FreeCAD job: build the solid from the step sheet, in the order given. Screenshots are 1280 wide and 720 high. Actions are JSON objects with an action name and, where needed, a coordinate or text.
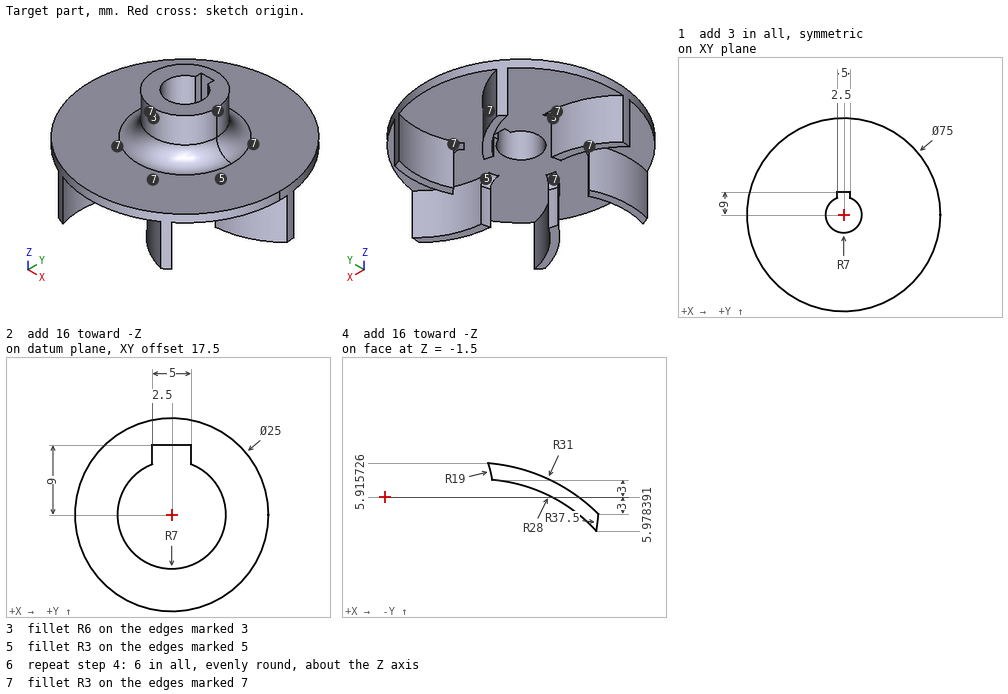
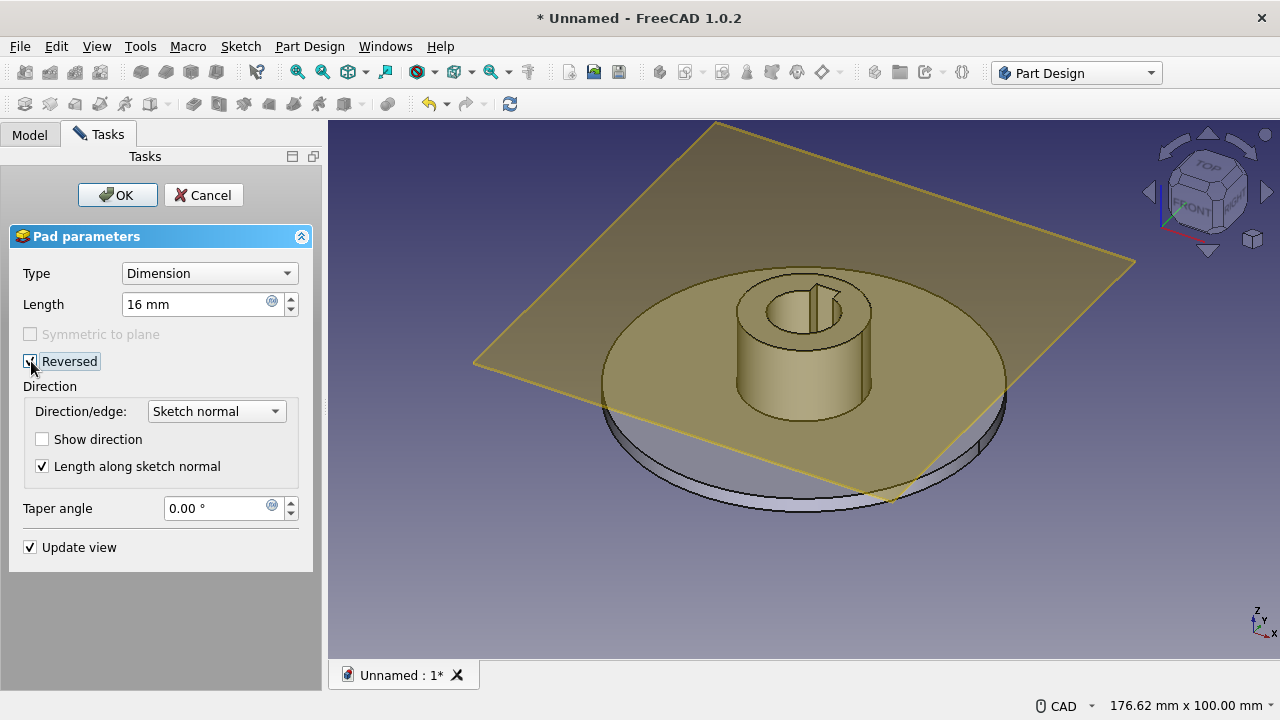
{"action": "left_click", "coordinate": [118, 195]}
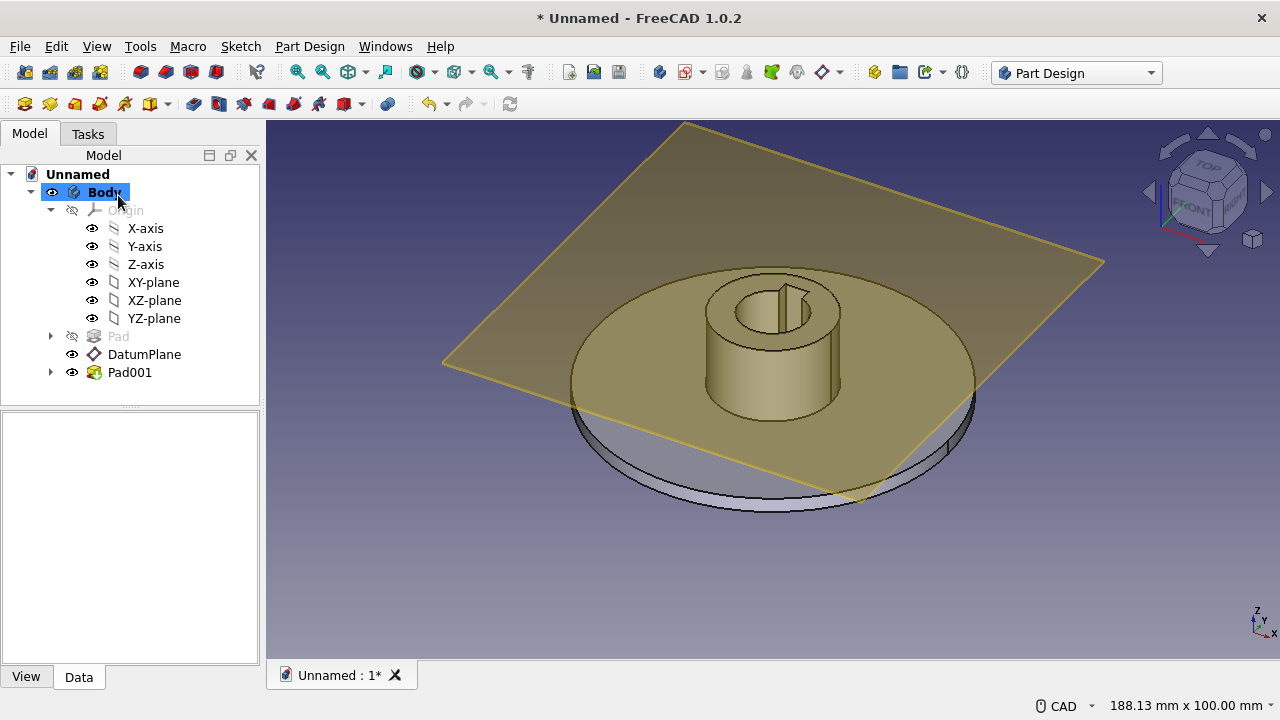
{"action": "left_click", "coordinate": [117, 354]}
{"action": "key", "text": "space"}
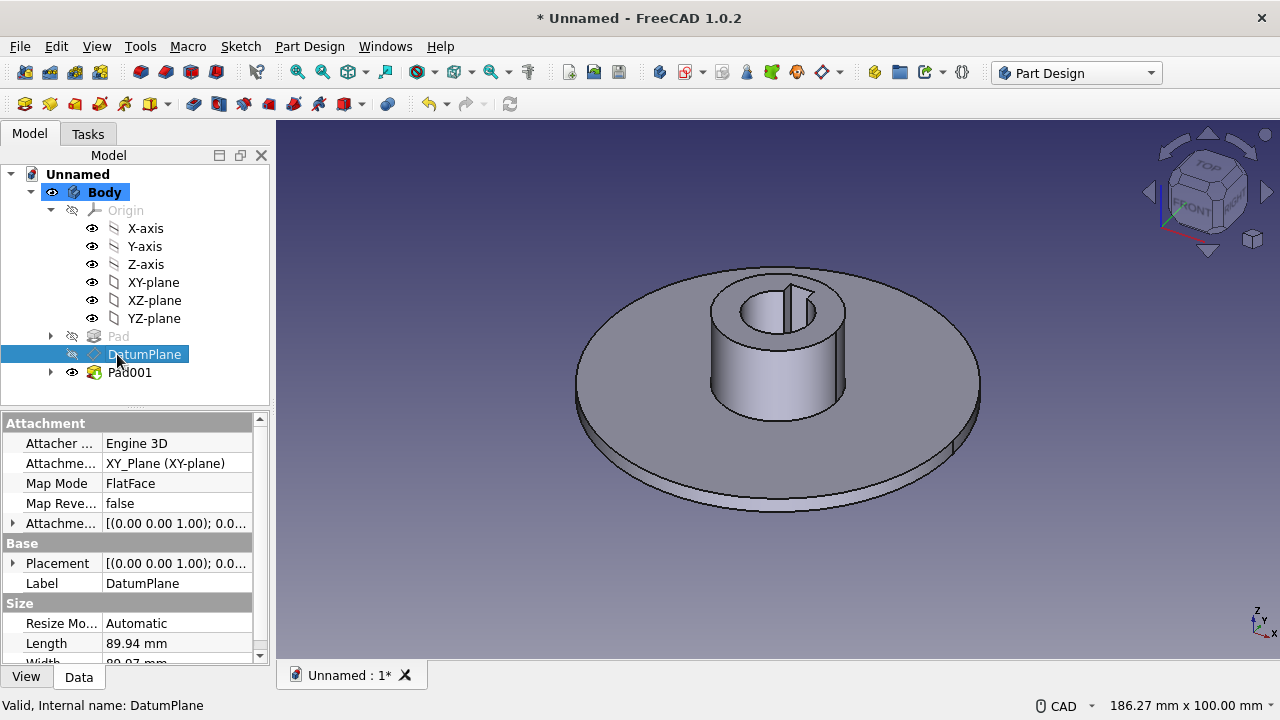
{"action": "key", "text": "0"}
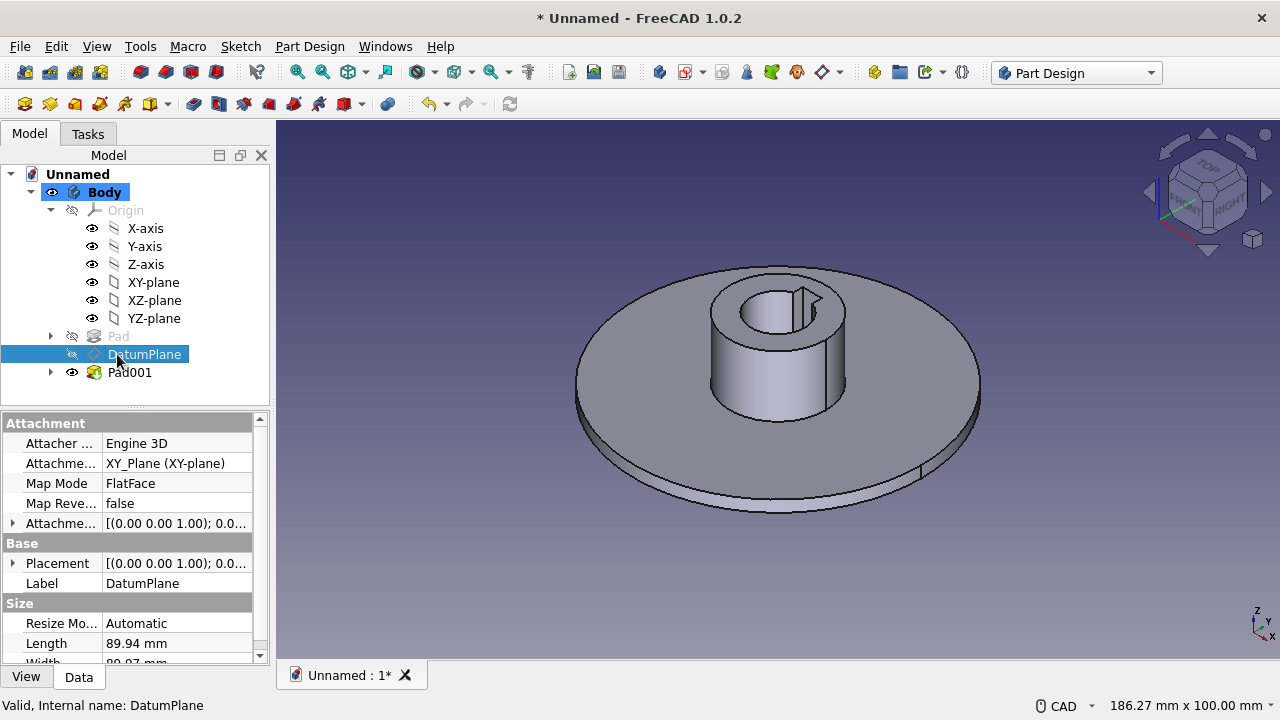
{"action": "key", "text": "2"}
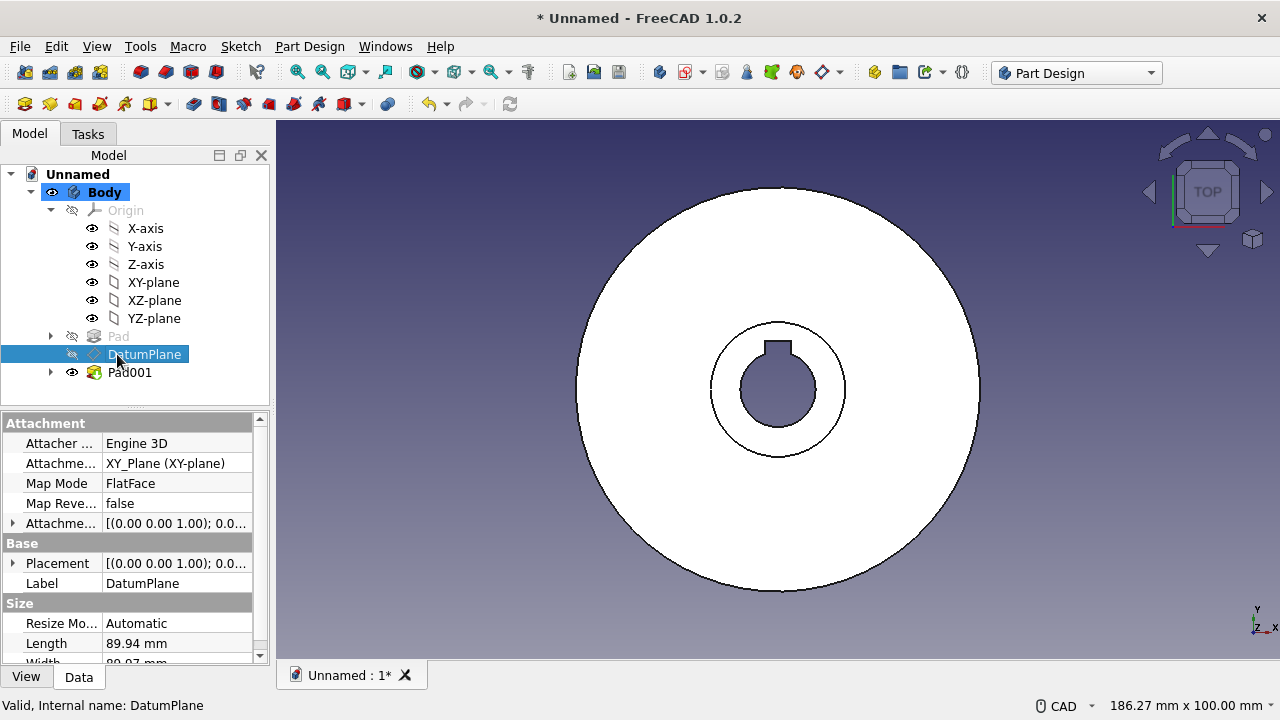
{"action": "key", "text": "1"}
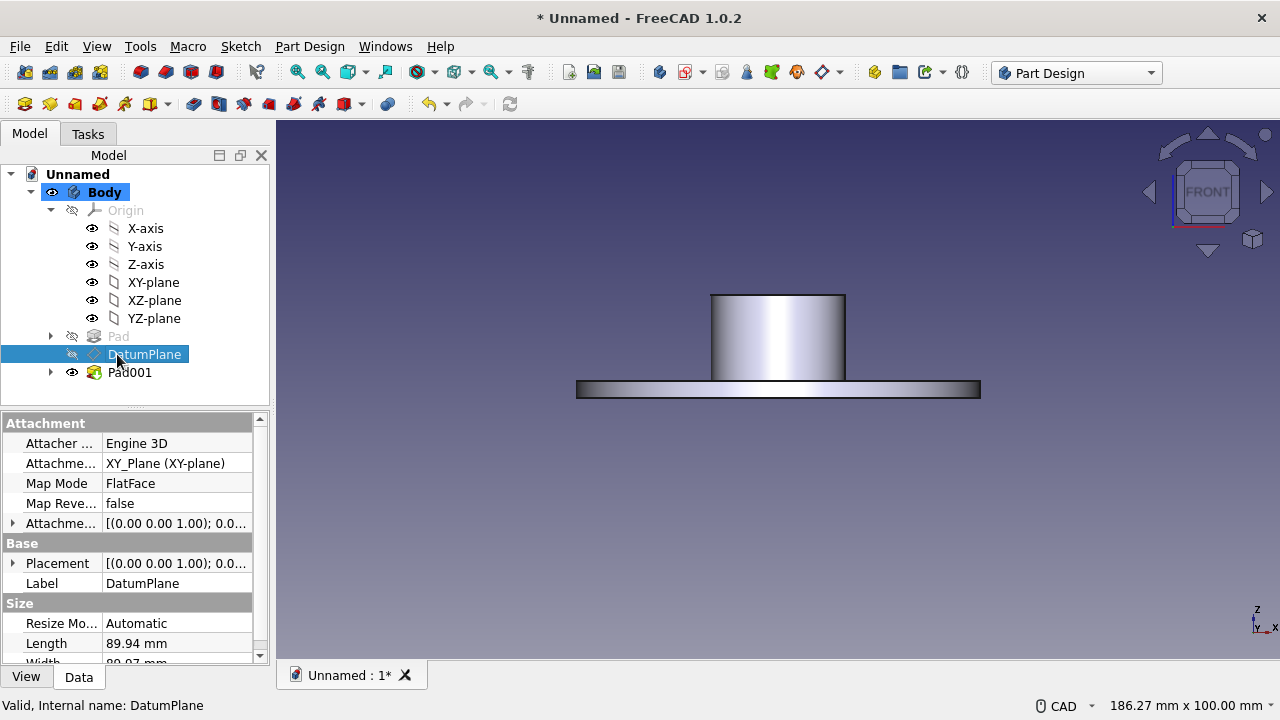
{"action": "left_click", "coordinate": [298, 72]}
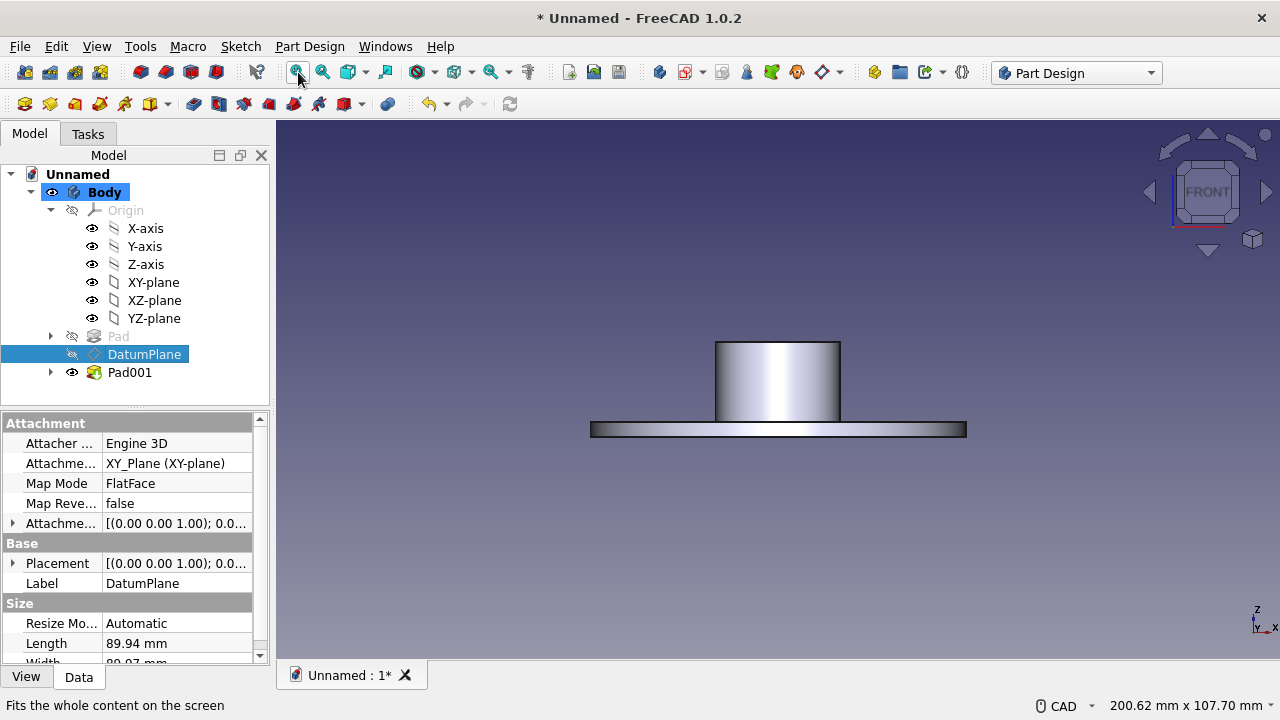
{"action": "key", "text": "3"}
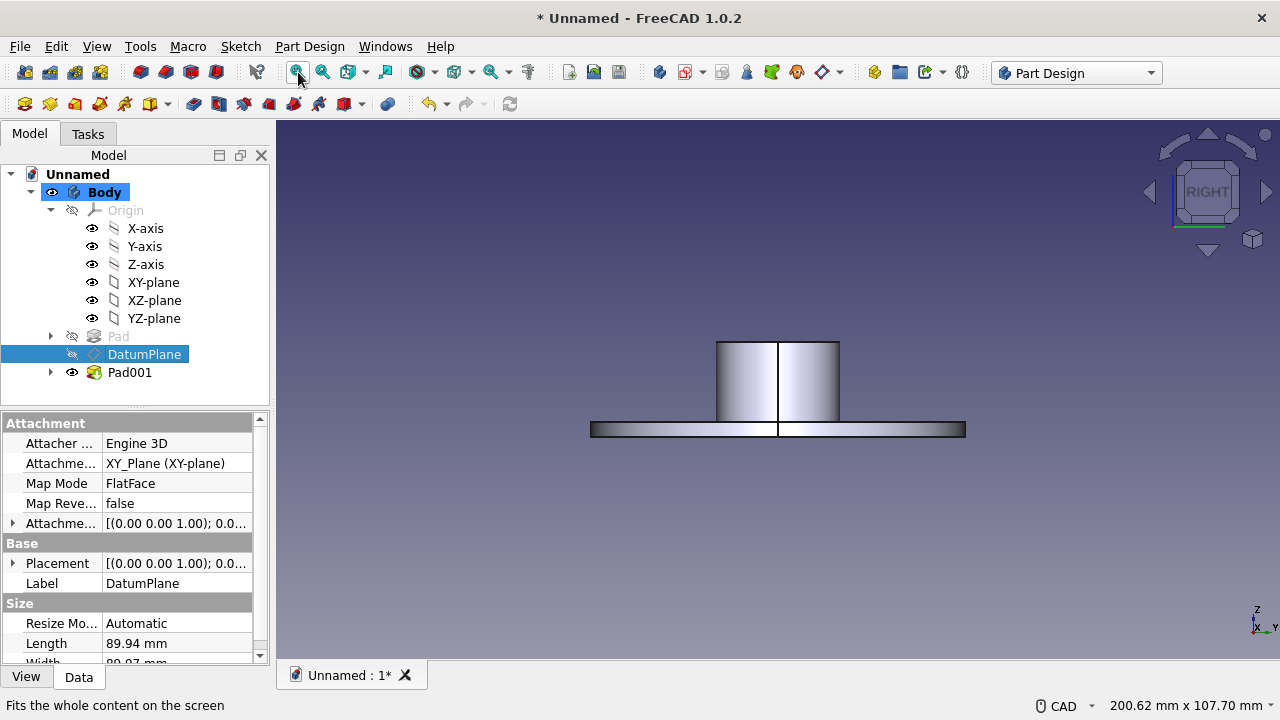
{"action": "left_click", "coordinate": [298, 72]}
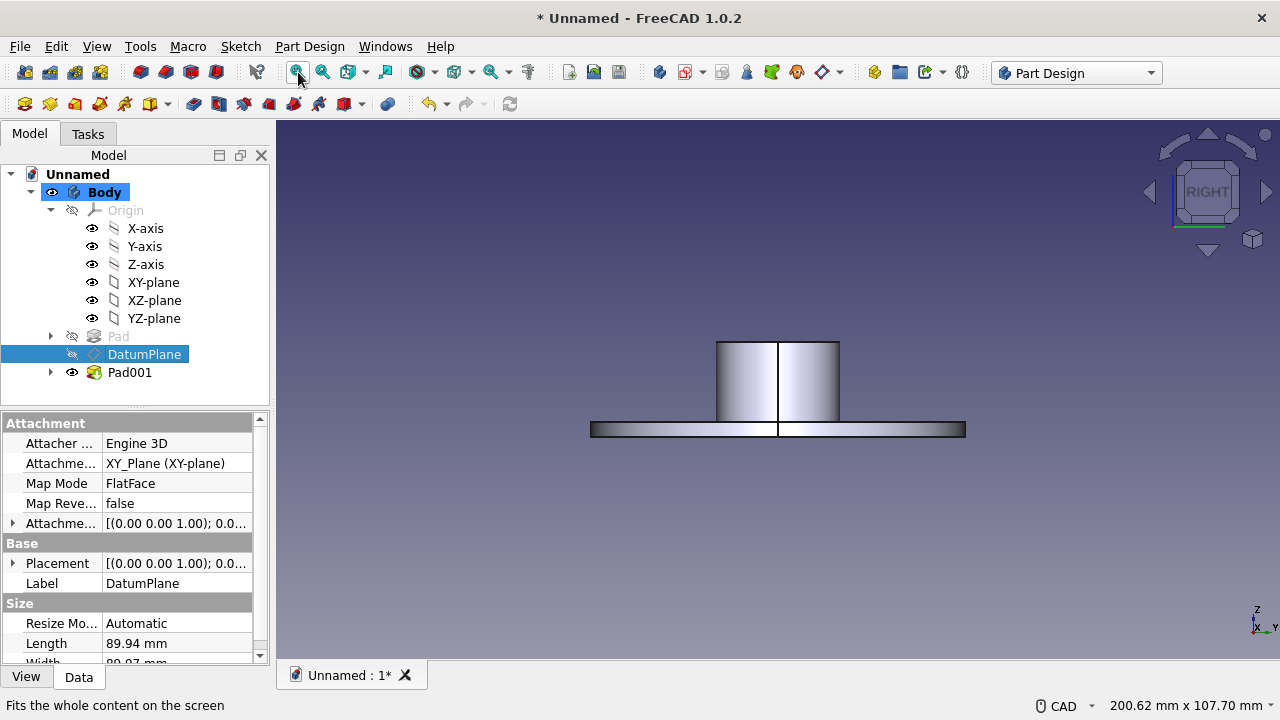
{"action": "key", "text": "5"}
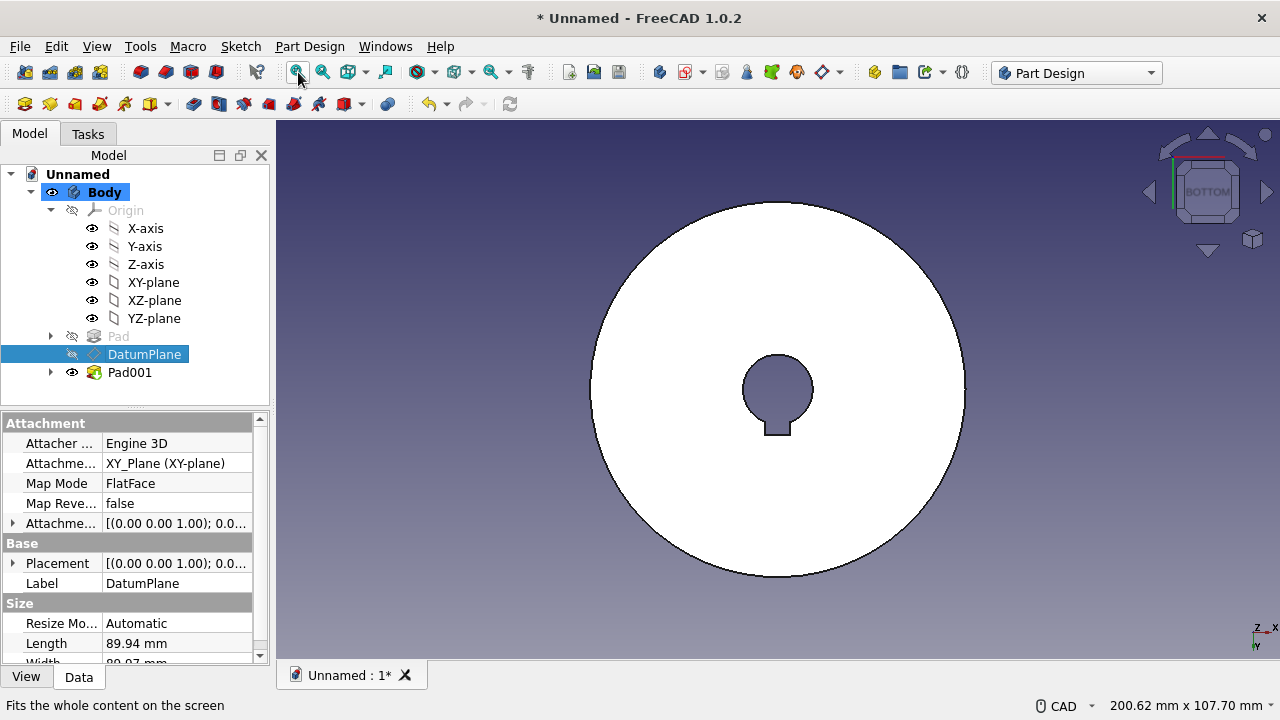
{"action": "key", "text": "4"}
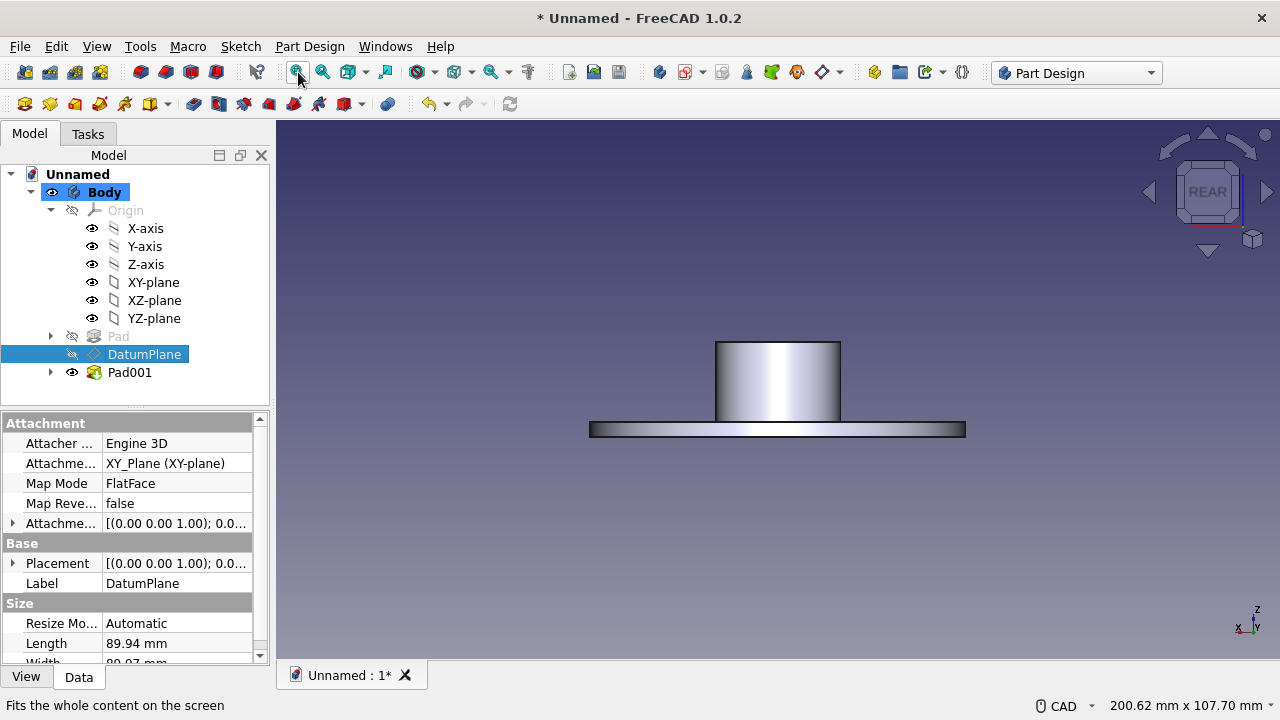
{"action": "left_click", "coordinate": [298, 72]}